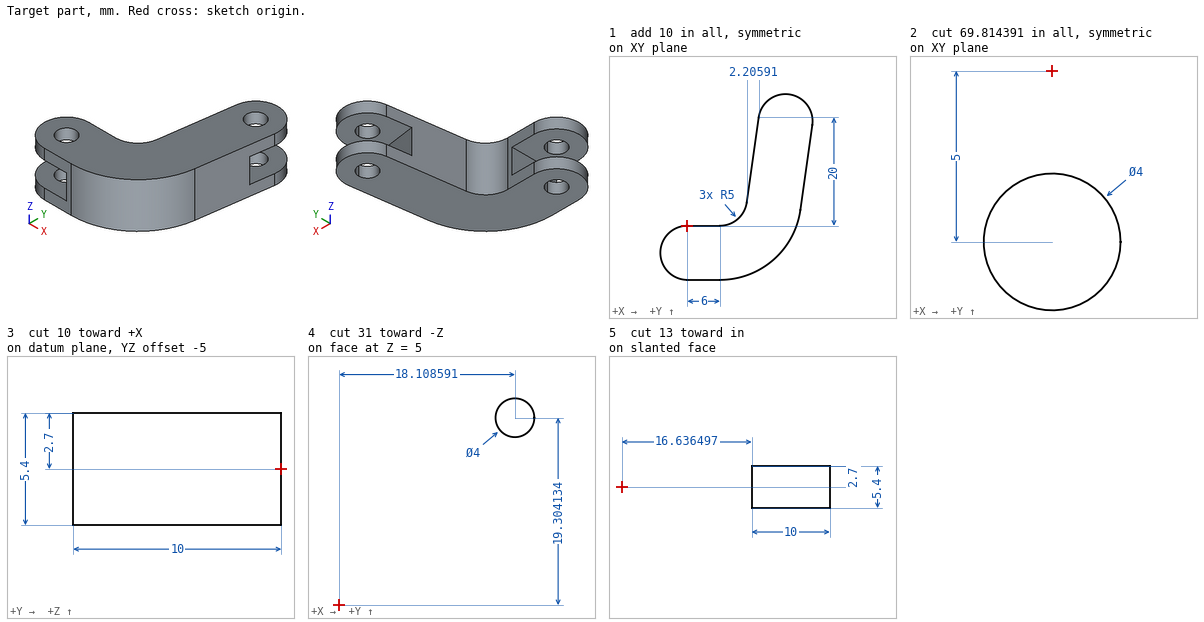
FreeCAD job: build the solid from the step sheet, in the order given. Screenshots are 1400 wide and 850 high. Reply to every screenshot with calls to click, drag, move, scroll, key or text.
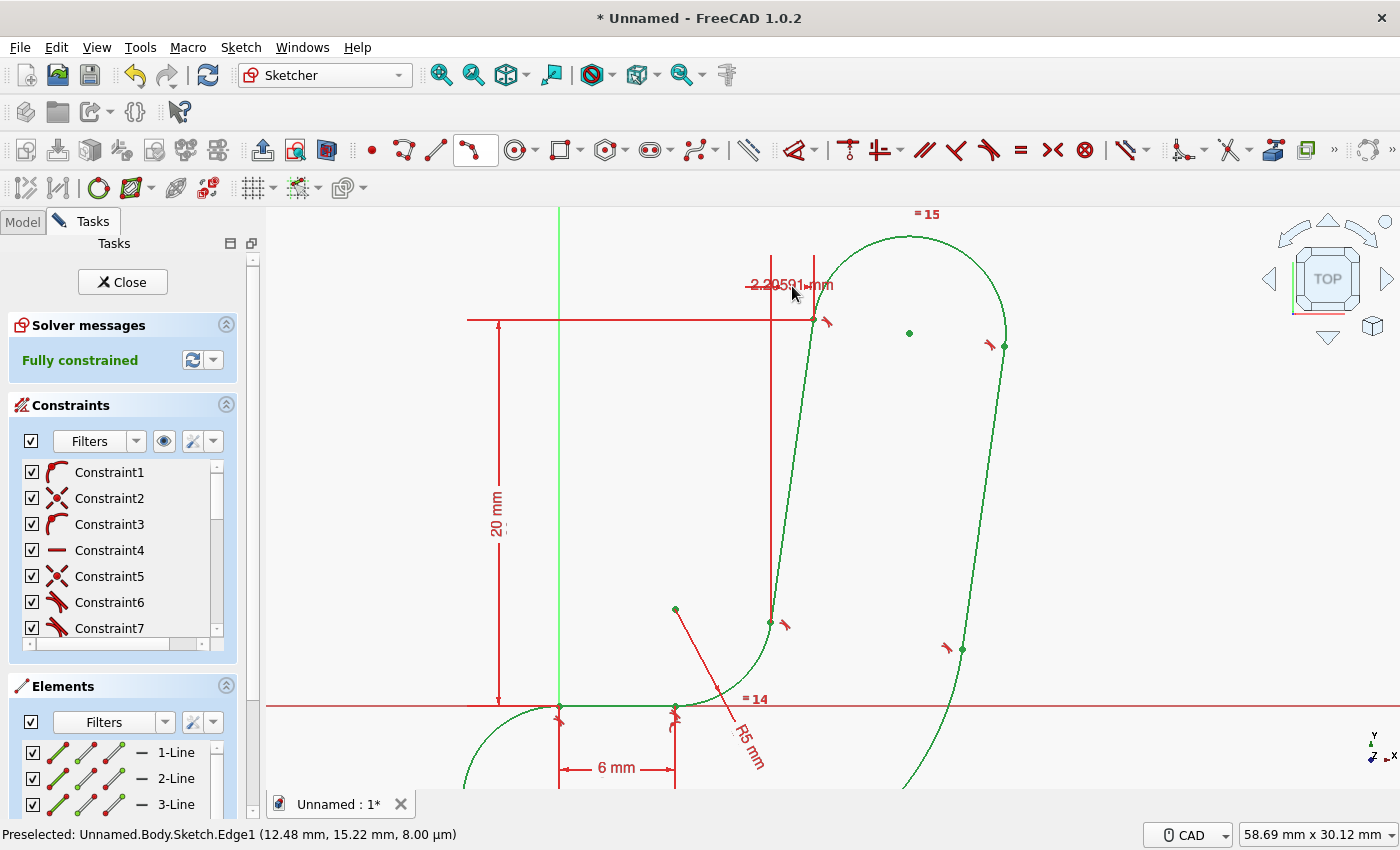
click(123, 282)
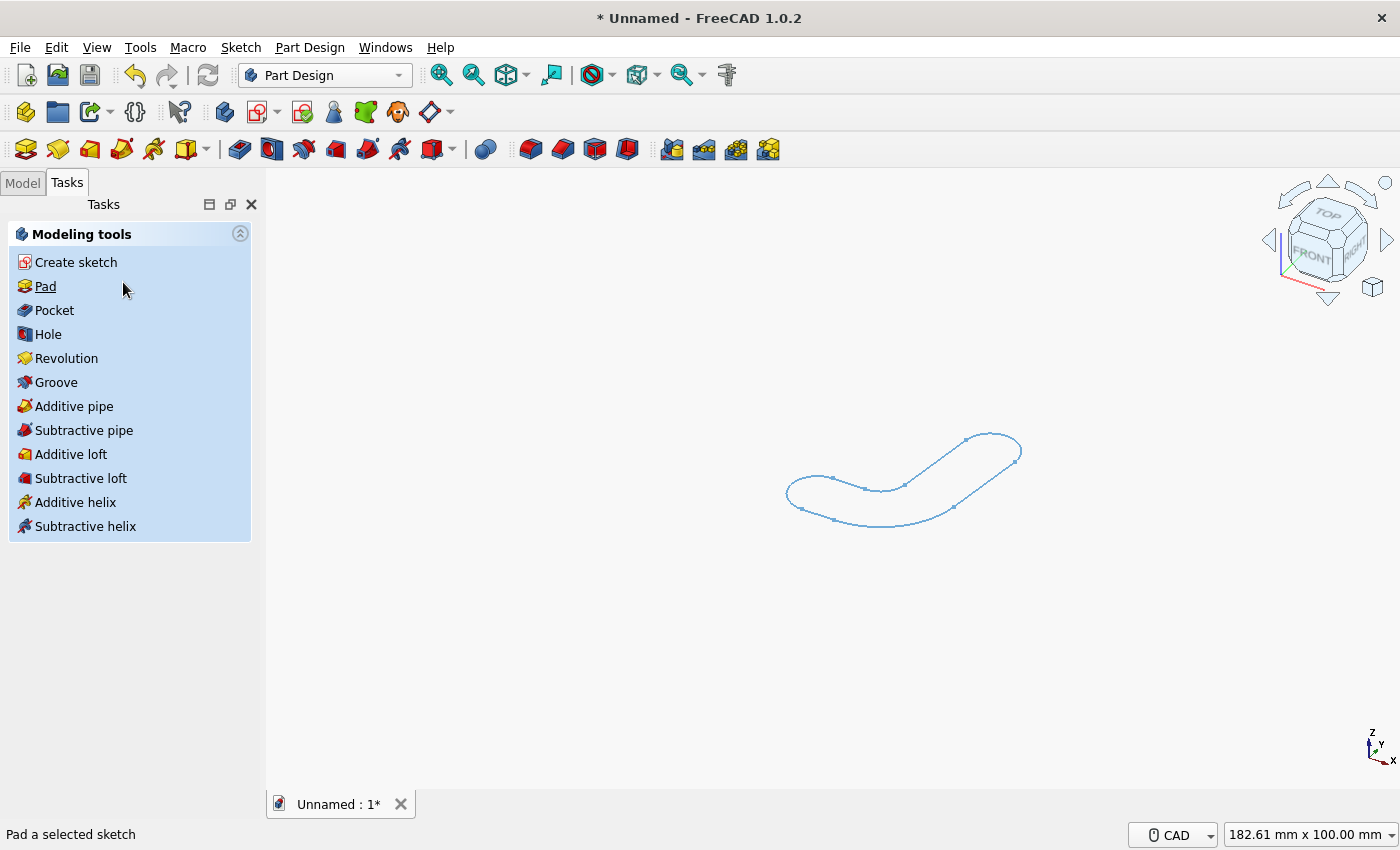
click(26, 150)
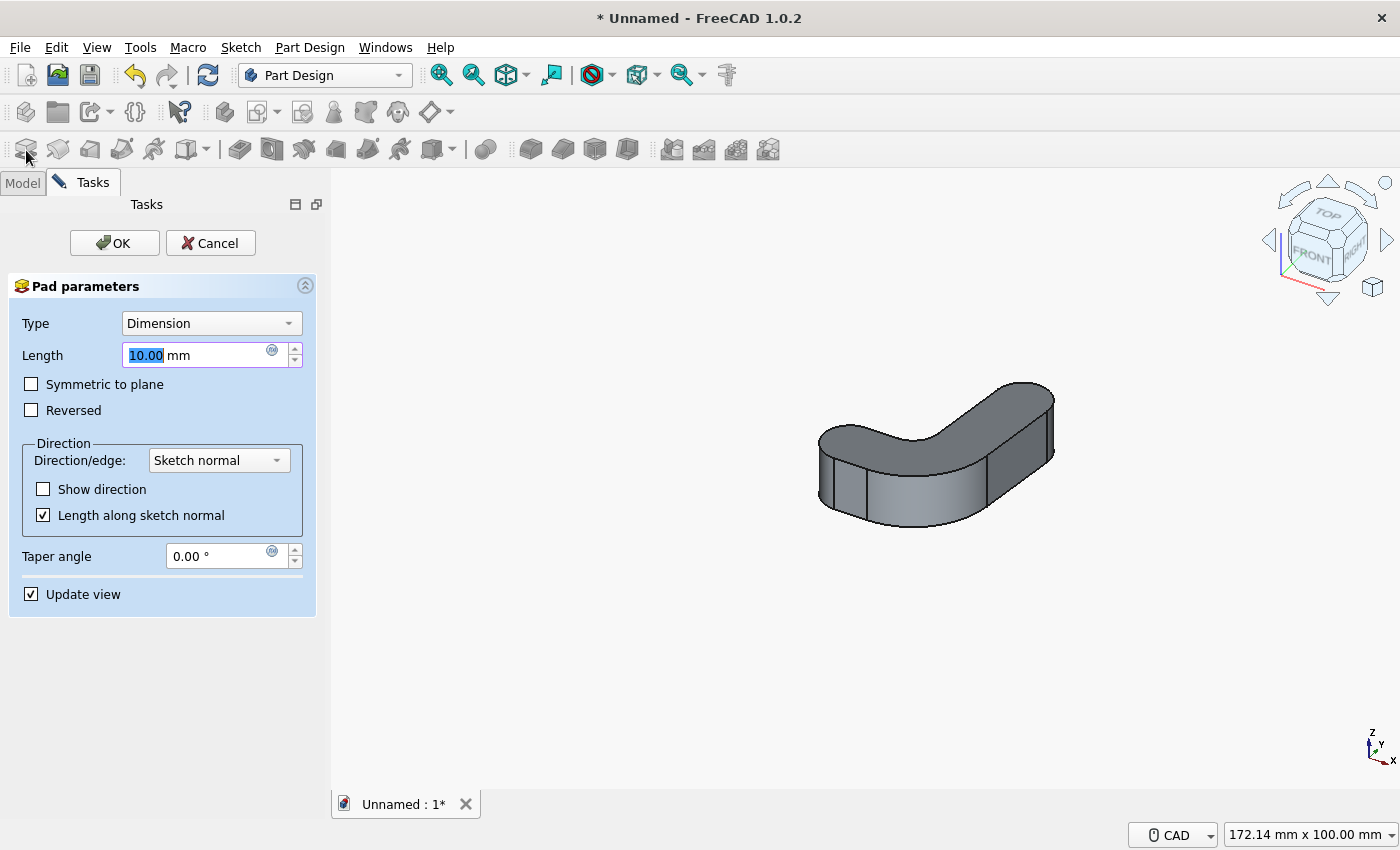
text(10)
key(Tab)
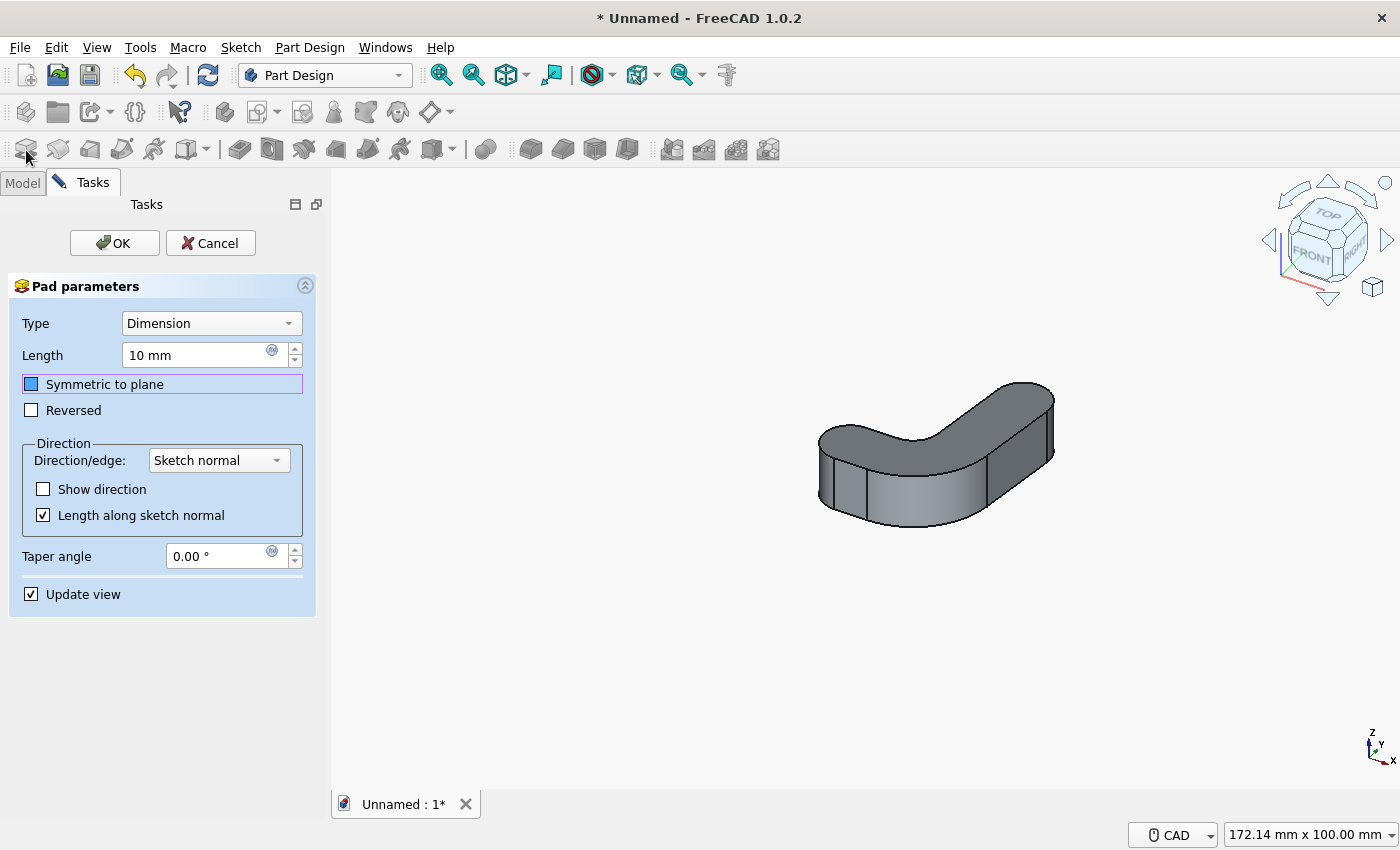
click(30, 384)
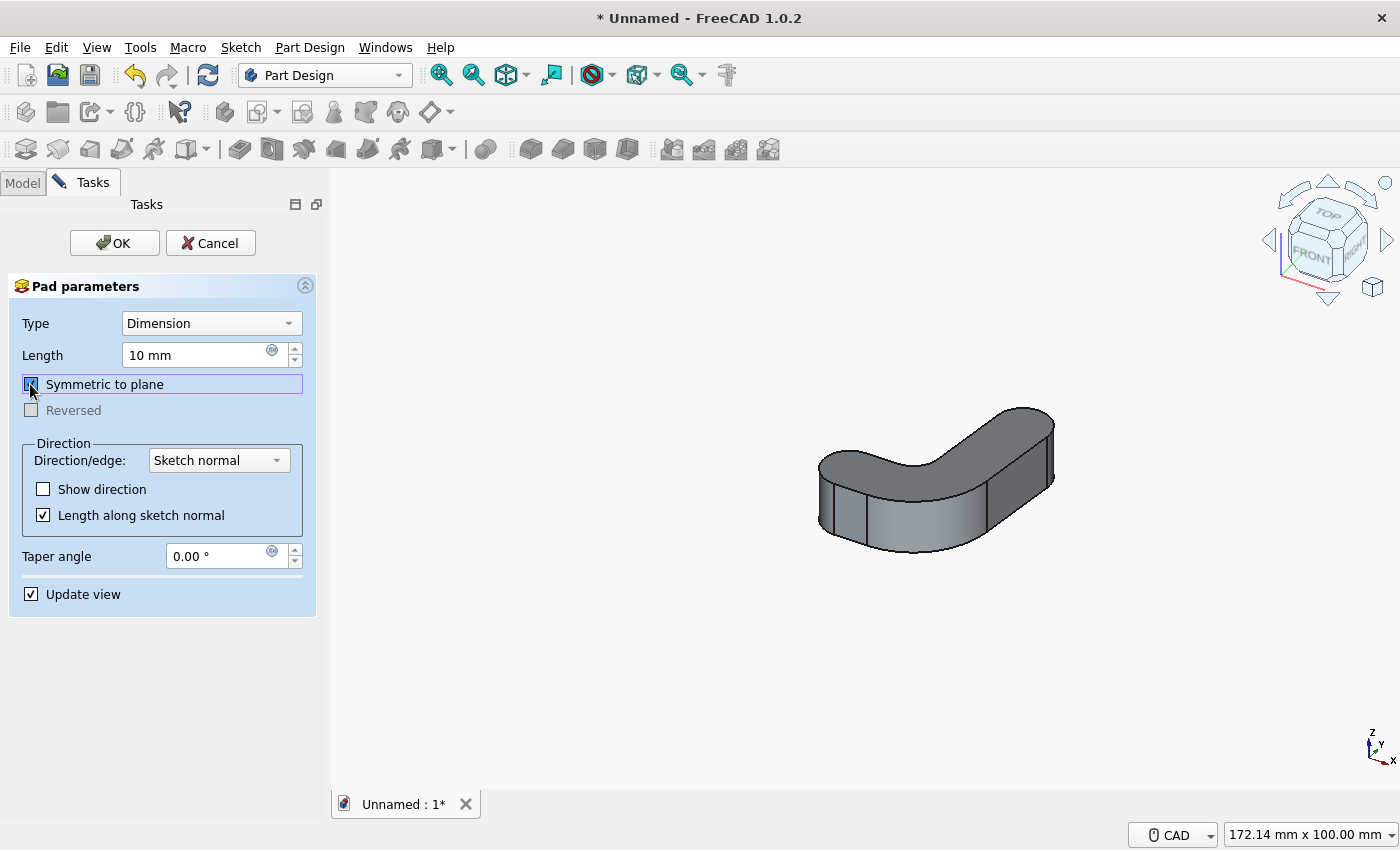
click(115, 243)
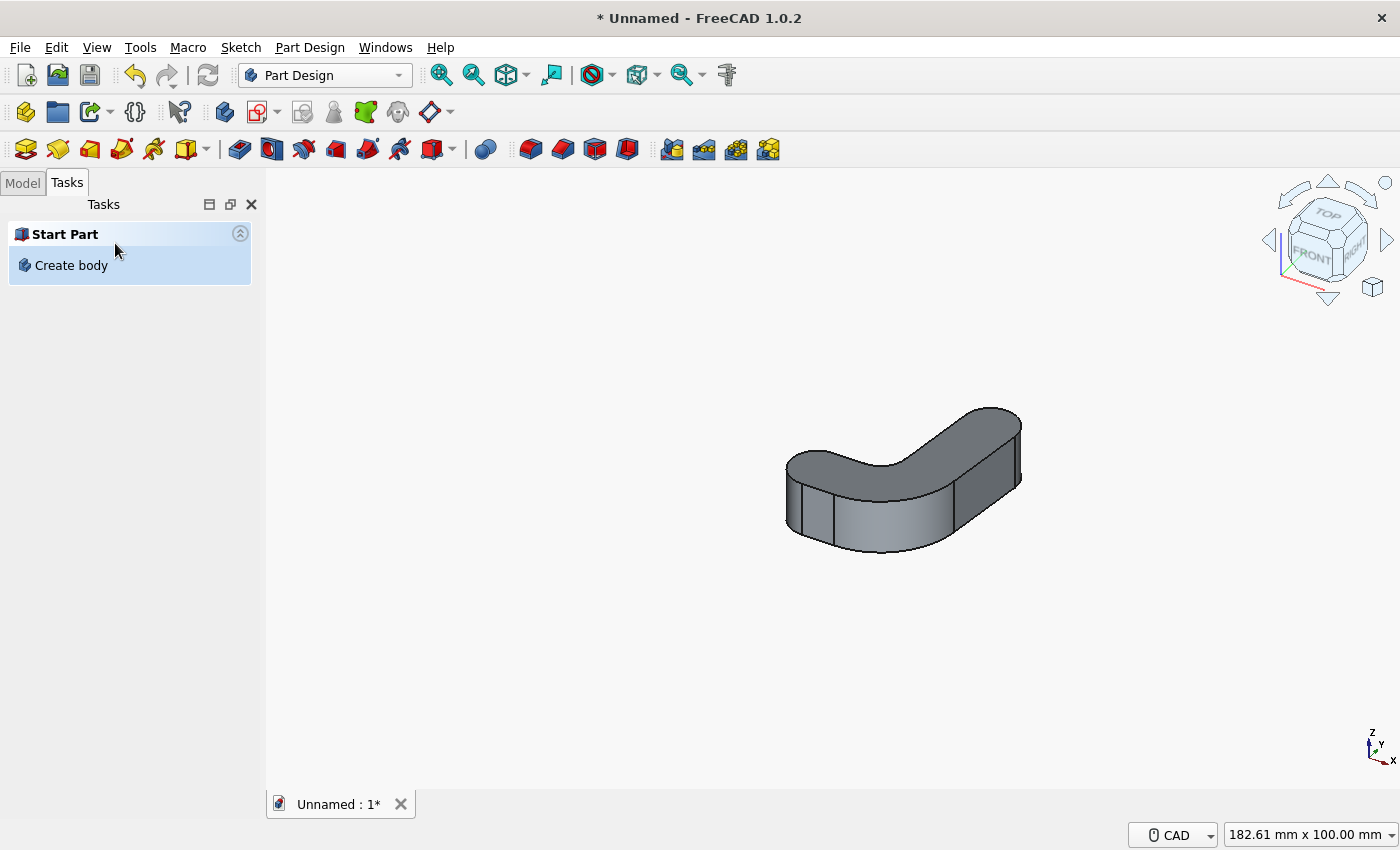
click(442, 76)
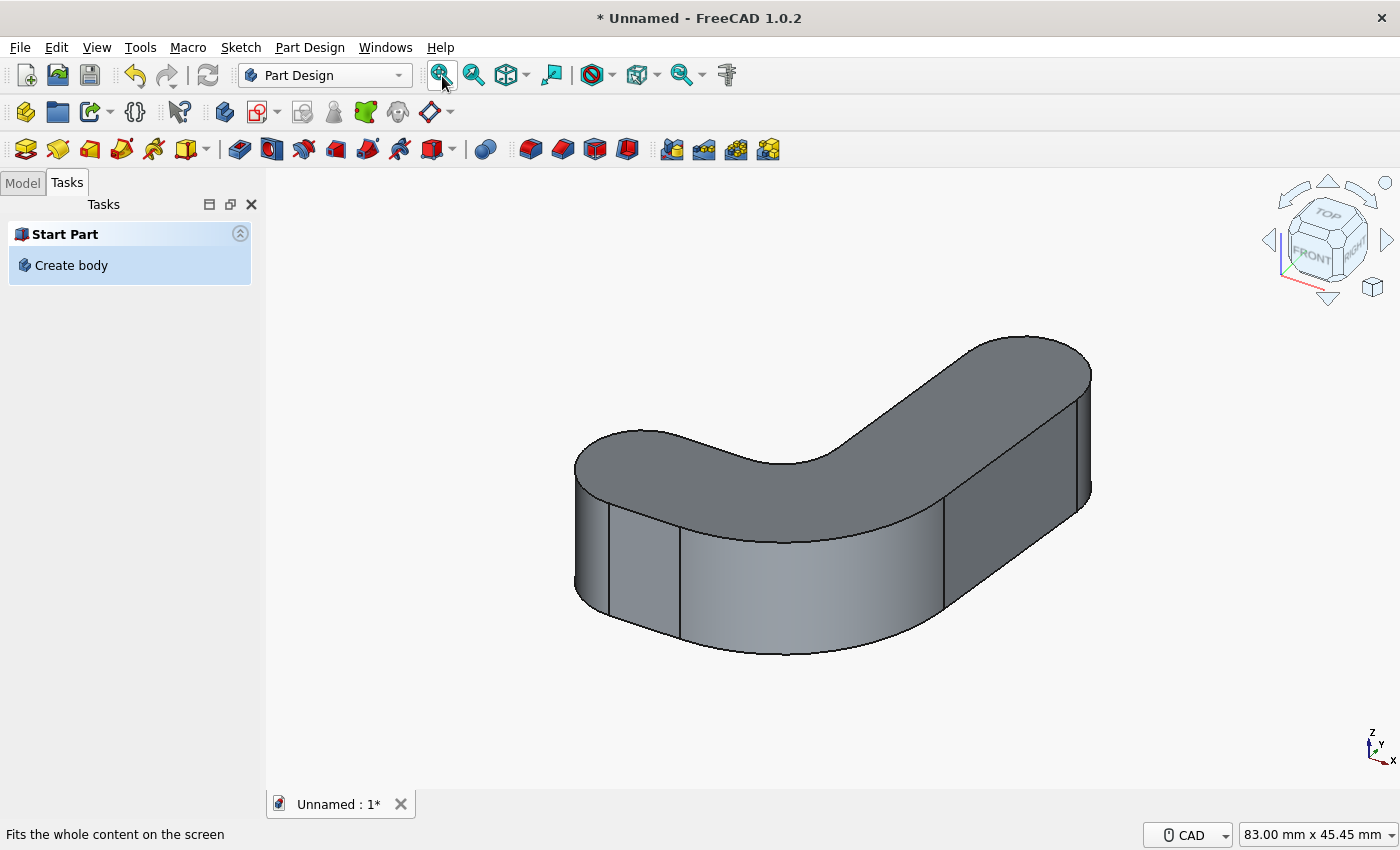
click(258, 112)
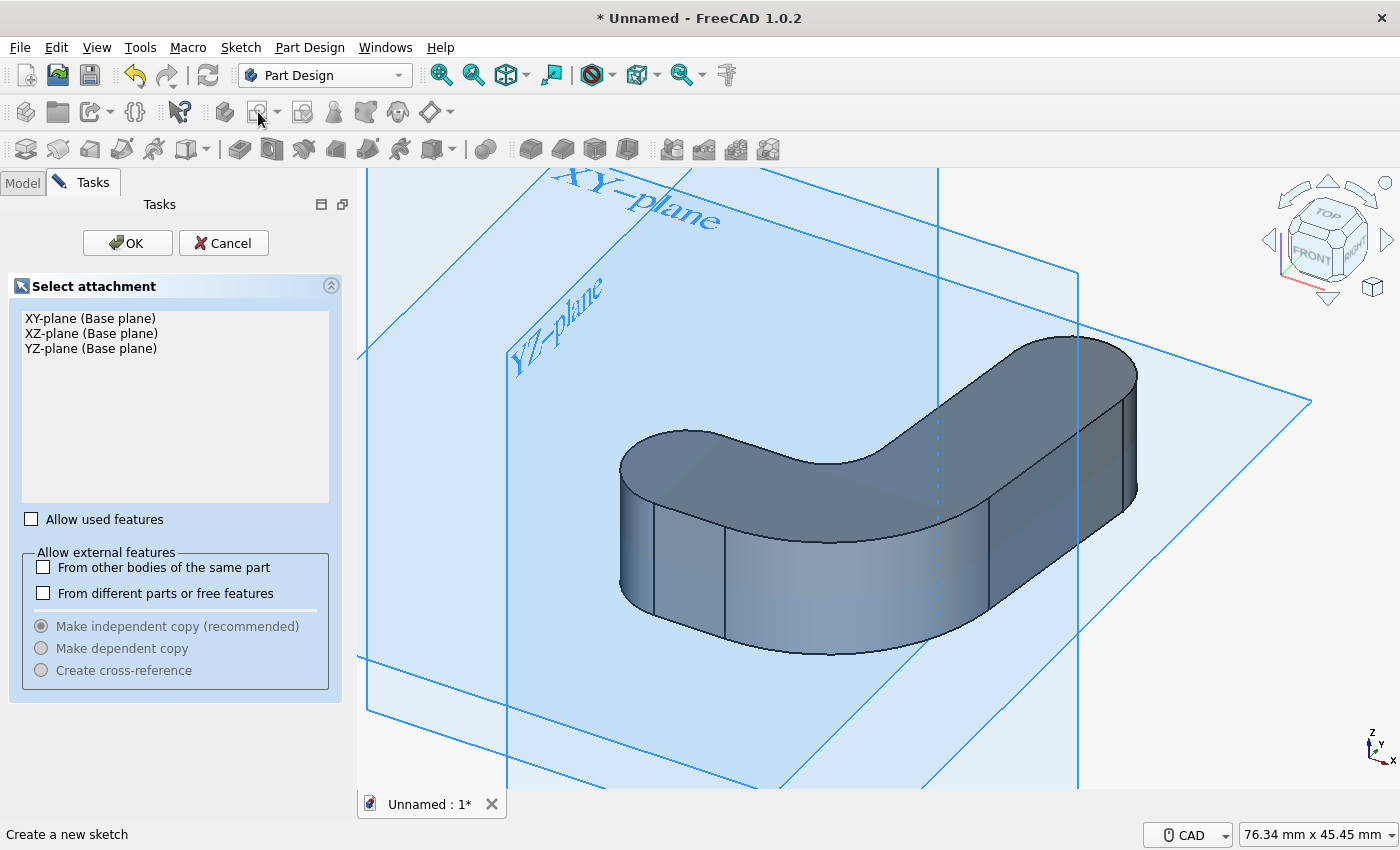
click(82, 318)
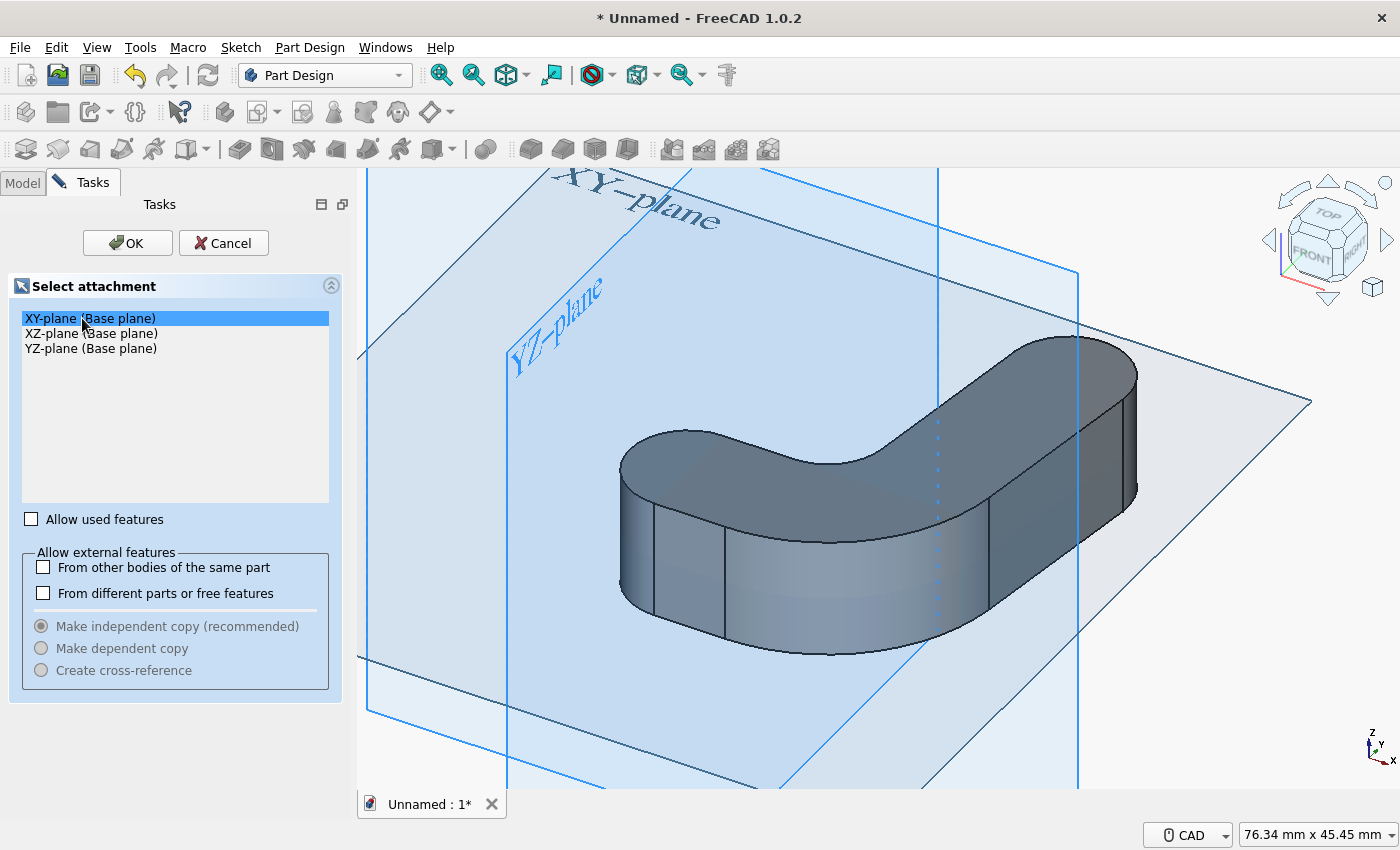
click(128, 243)